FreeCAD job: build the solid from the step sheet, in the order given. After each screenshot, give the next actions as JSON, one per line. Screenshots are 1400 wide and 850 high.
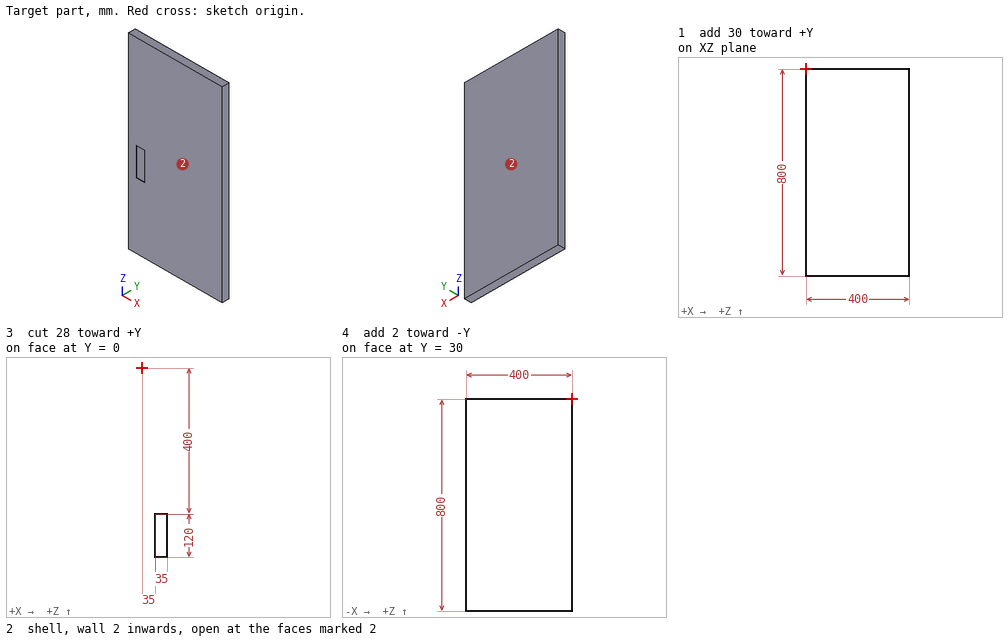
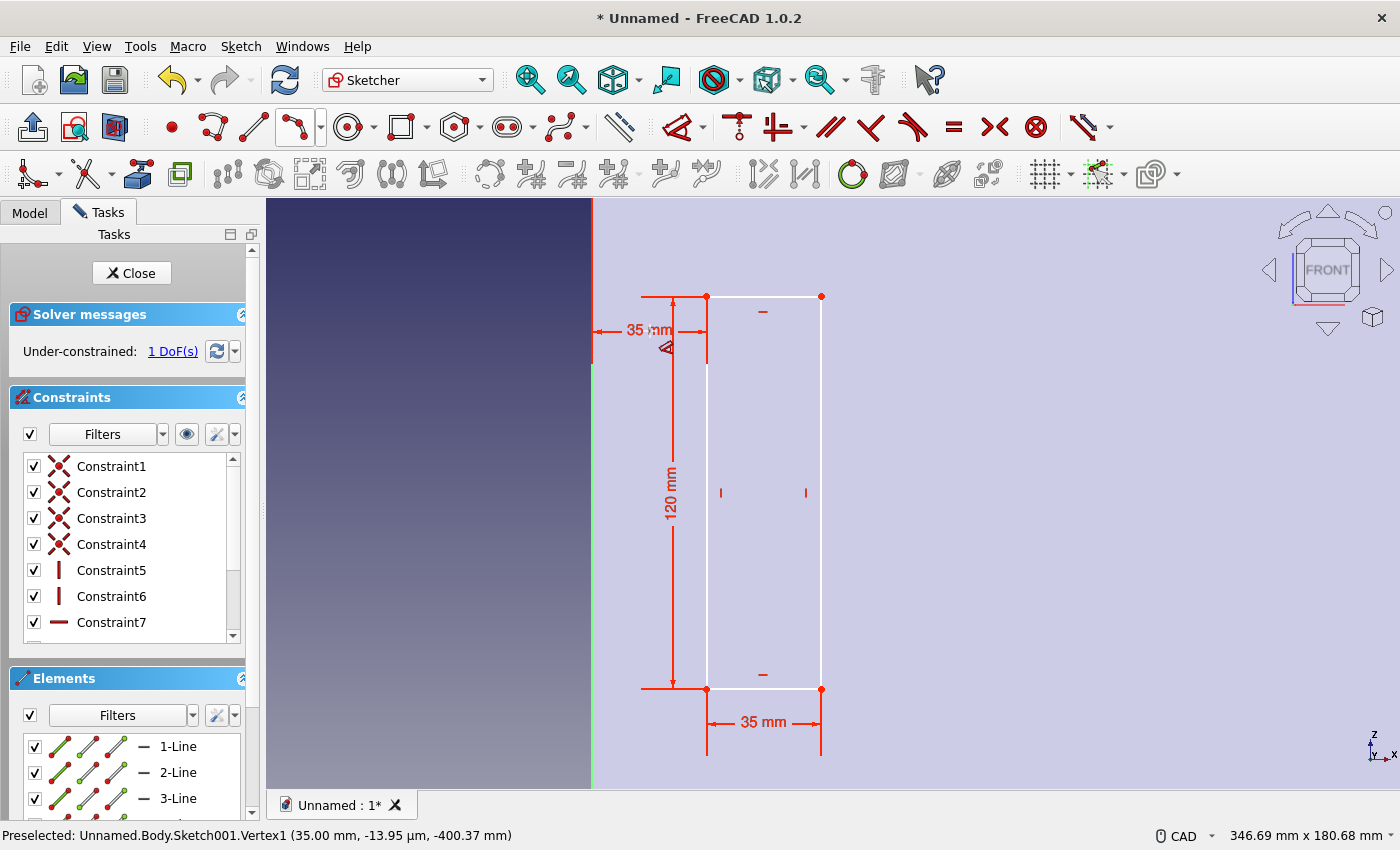
{"action": "left_click", "coordinate": [707, 297]}
{"action": "left_click", "coordinate": [558, 261]}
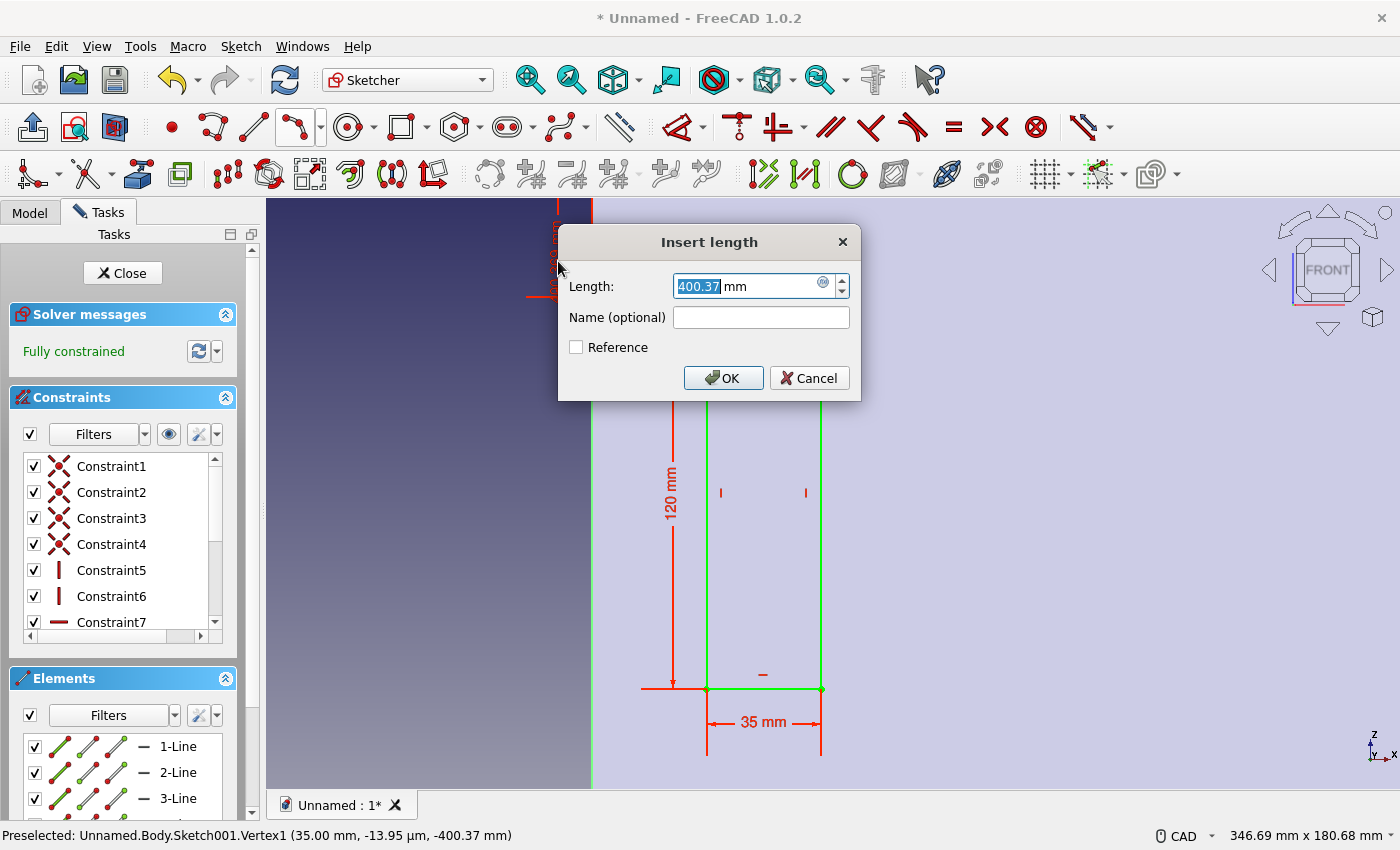
{"action": "type", "text": "400"}
{"action": "key", "text": "Return"}
{"action": "key", "text": "Escape"}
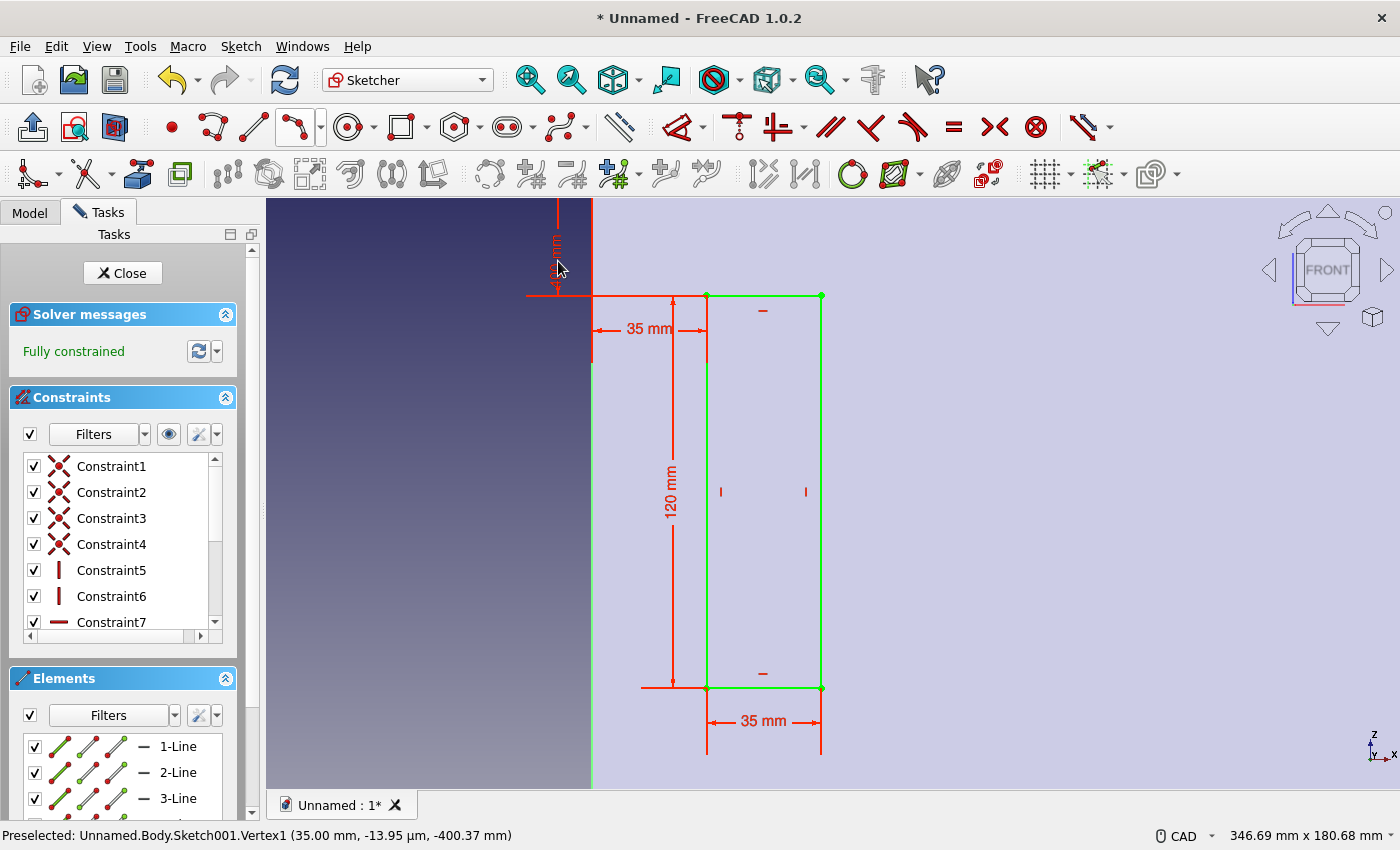
{"action": "left_click", "coordinate": [123, 273]}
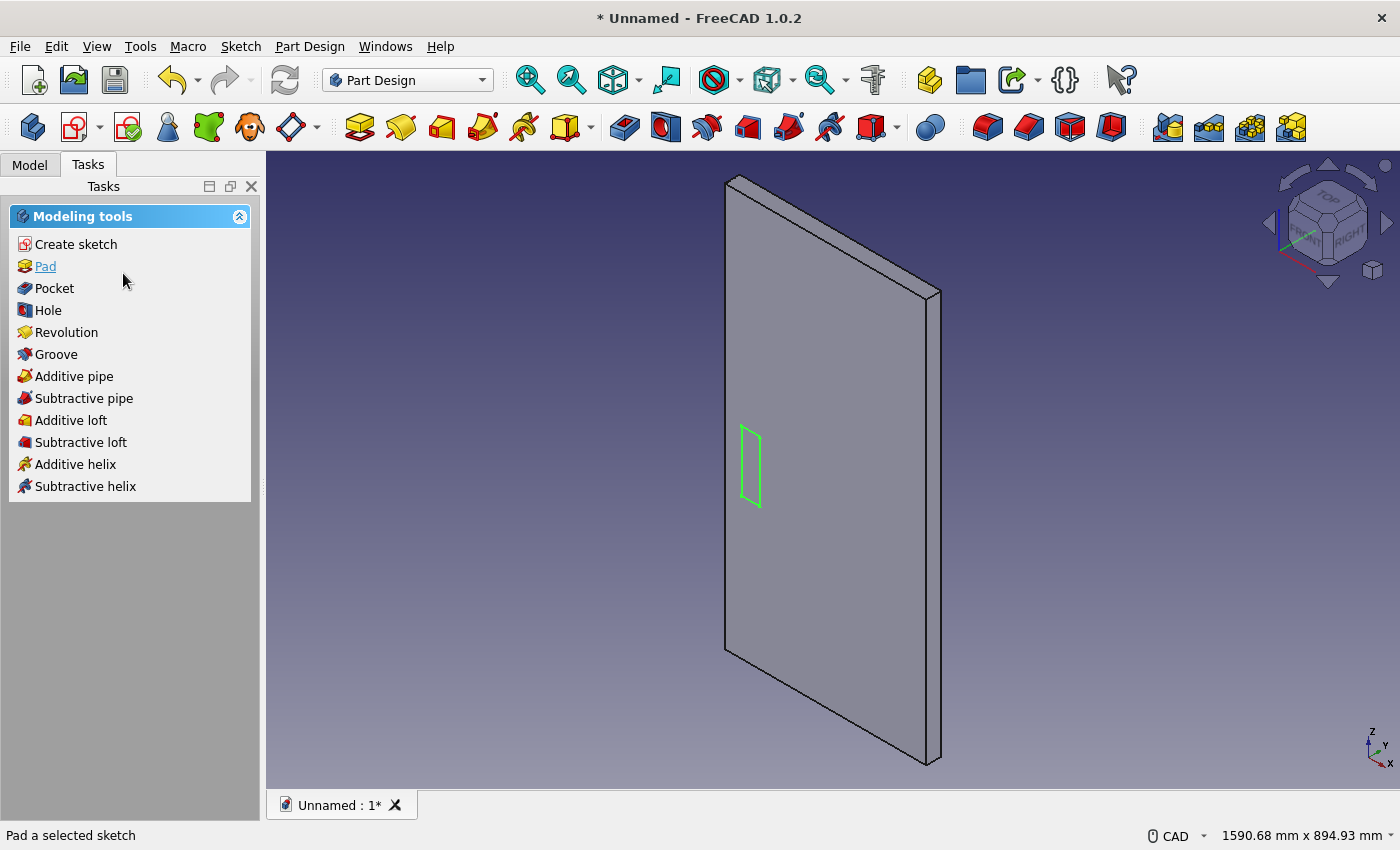
{"action": "left_click", "coordinate": [625, 128]}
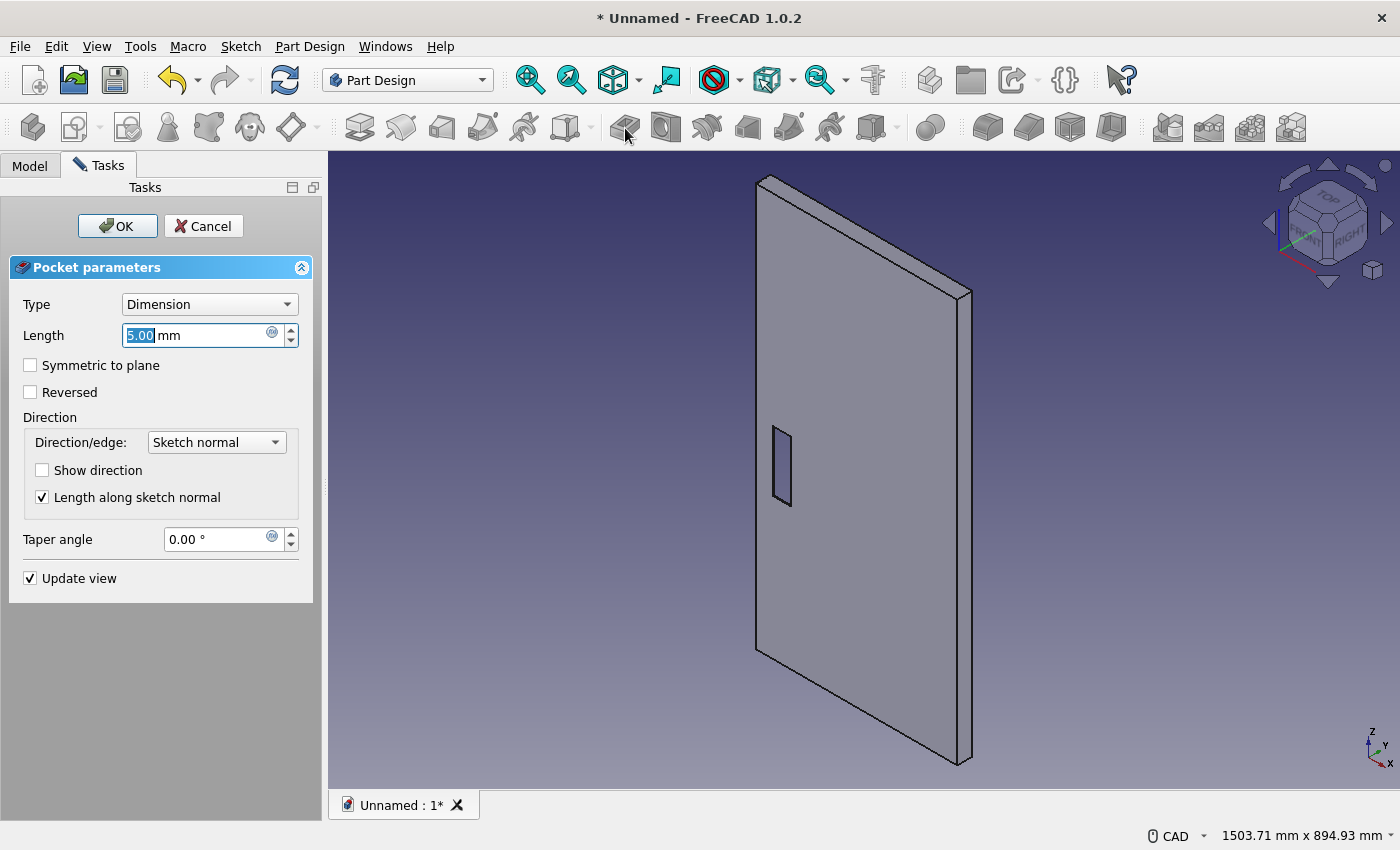
{"action": "type", "text": "28"}
{"action": "key", "text": "Tab"}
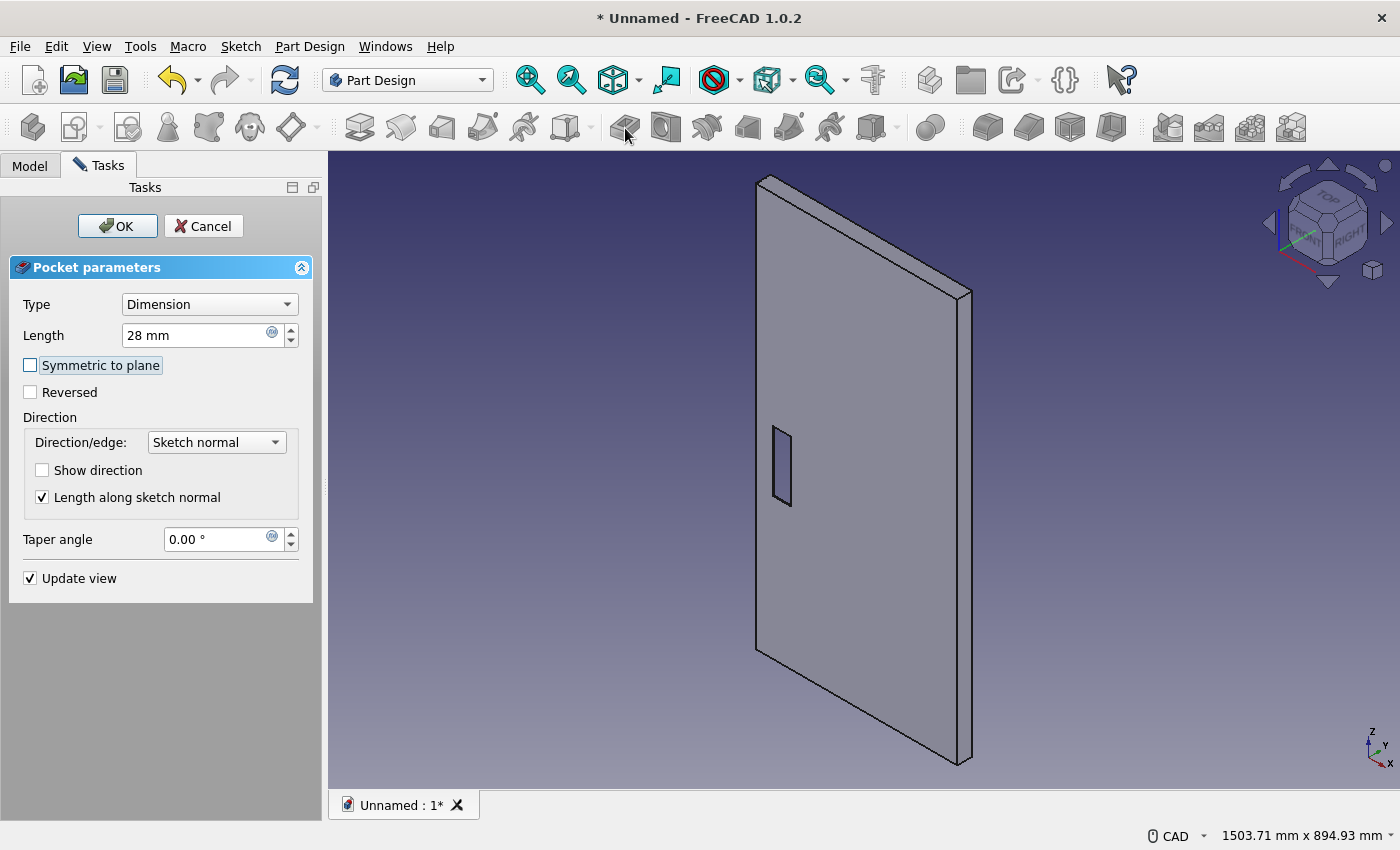
{"action": "left_click", "coordinate": [118, 226]}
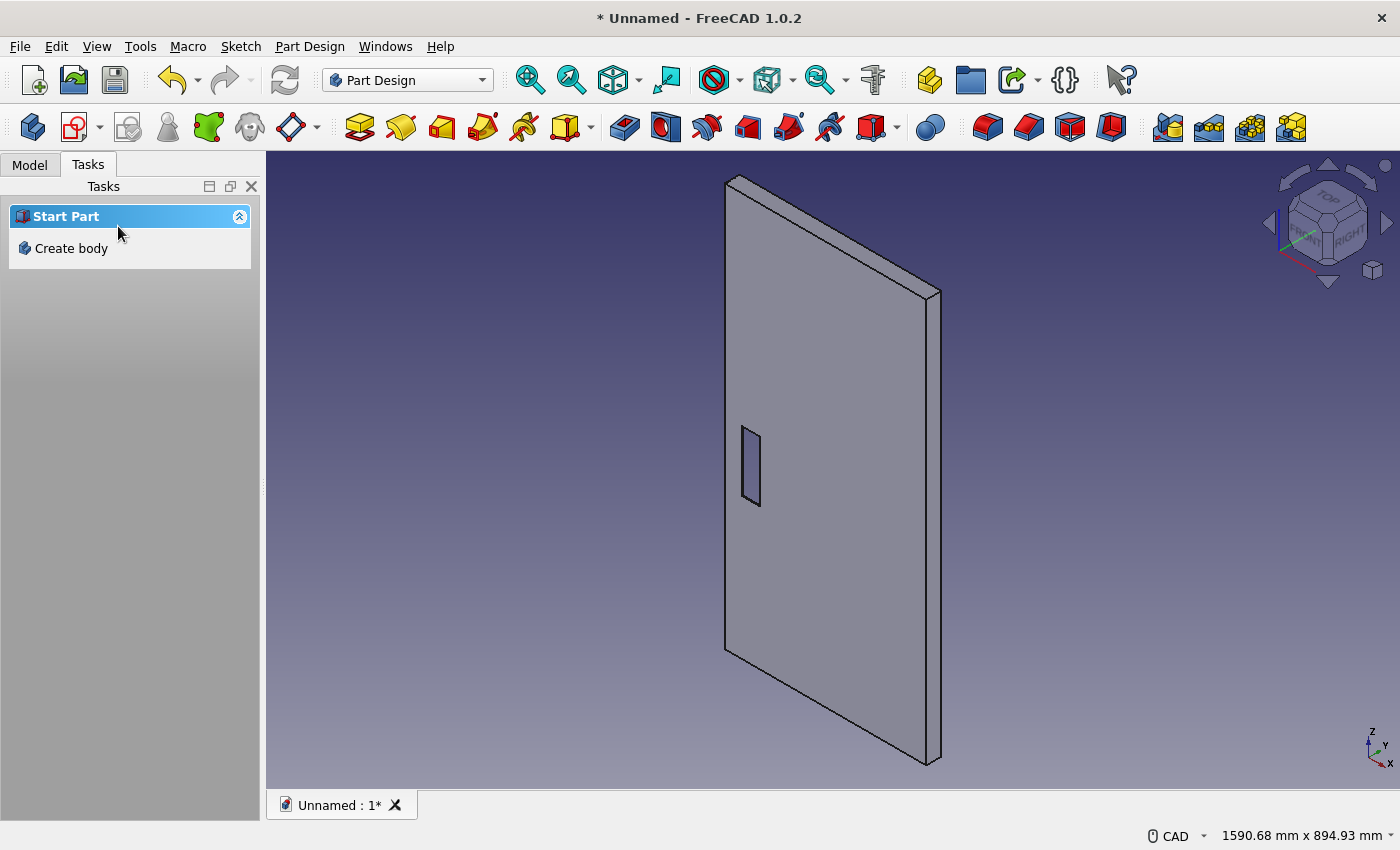
{"action": "key", "text": "4"}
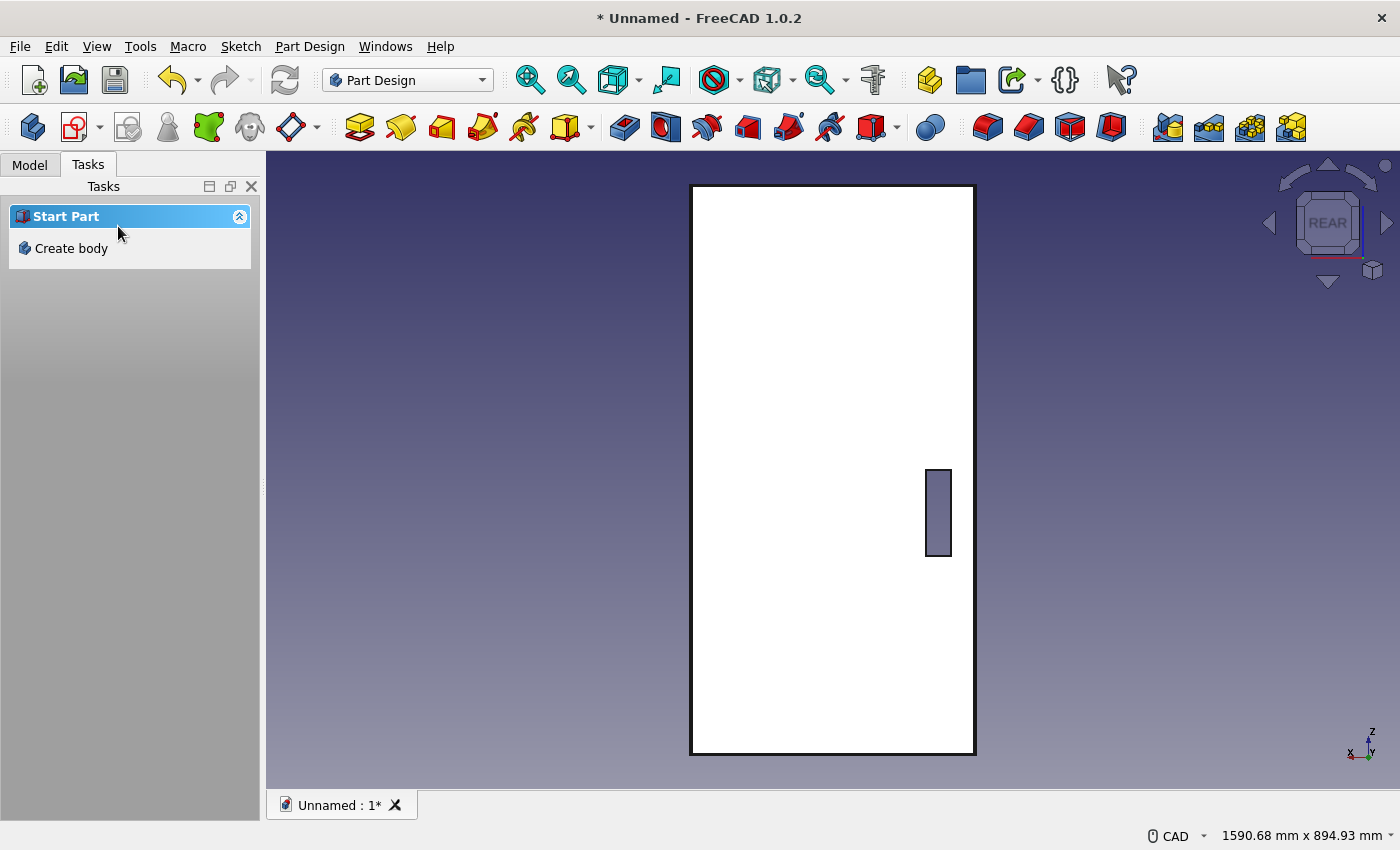
{"action": "scroll", "coordinate": [881, 753], "scroll_direction": "up", "scroll_amount": 15}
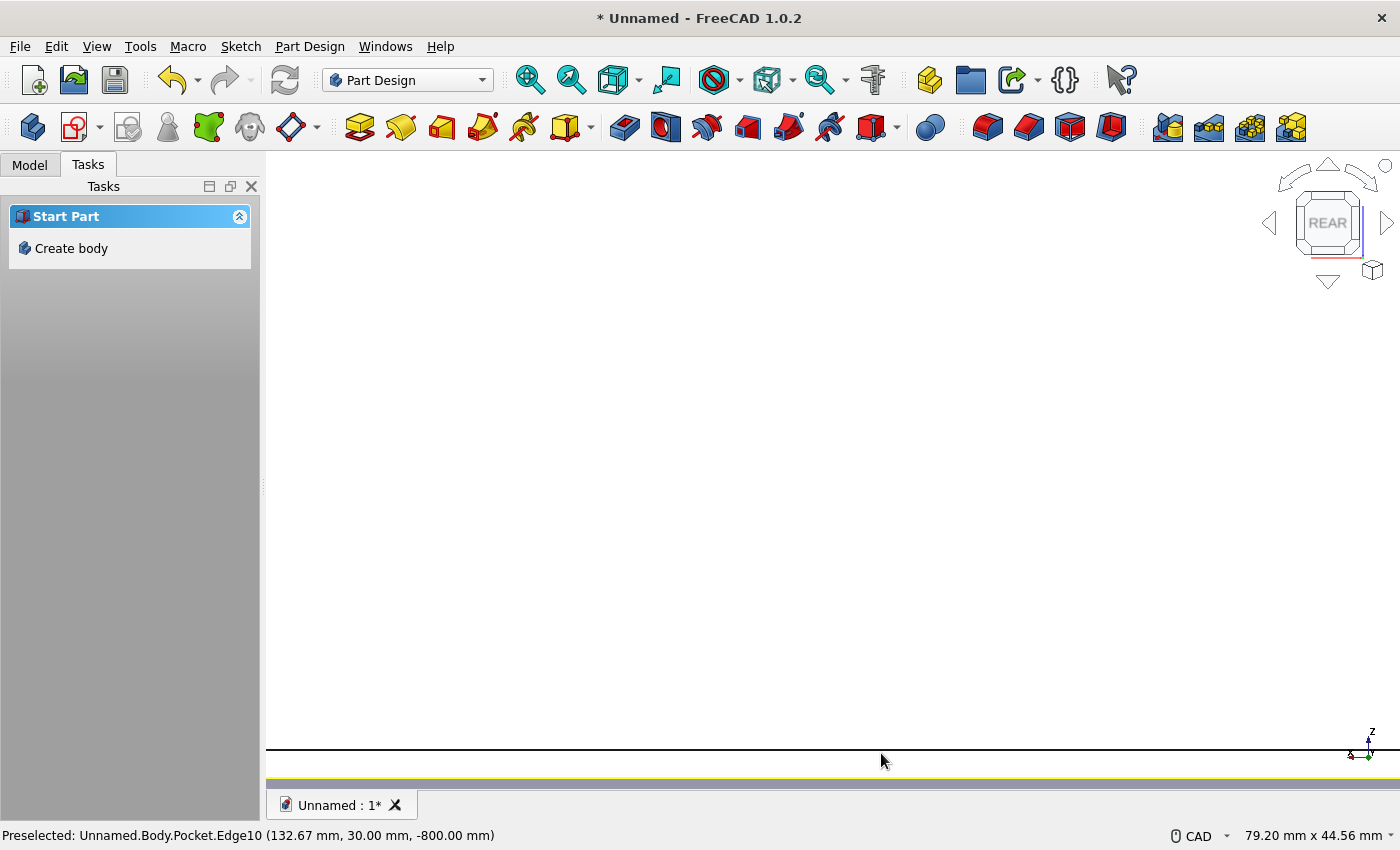
{"action": "left_click", "coordinate": [861, 758]}